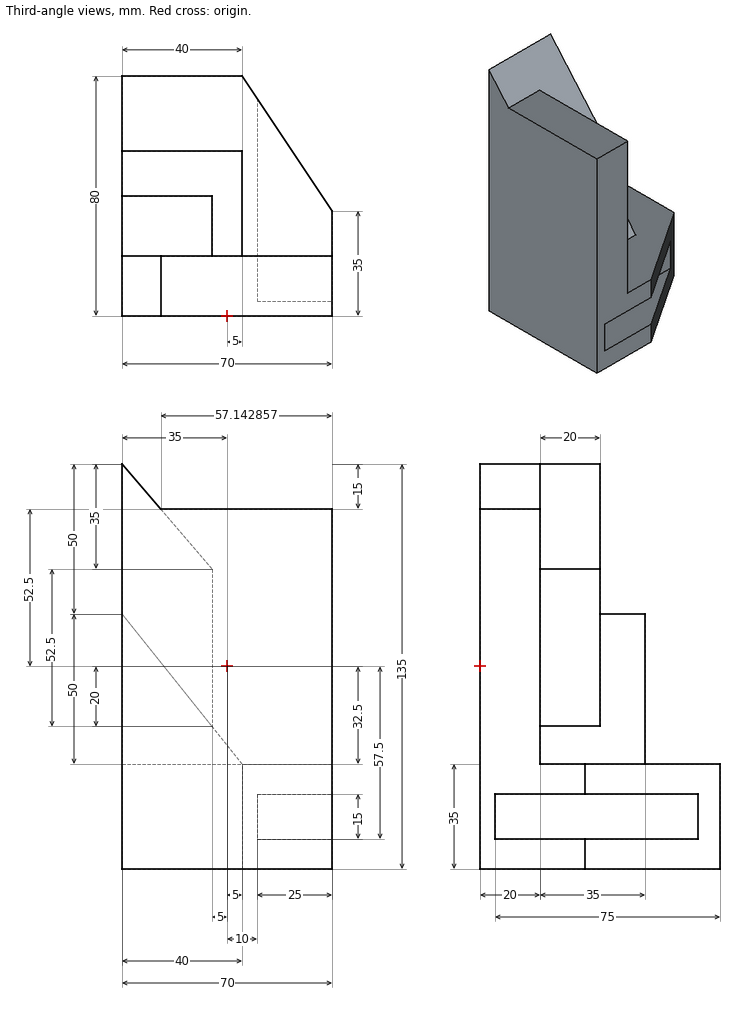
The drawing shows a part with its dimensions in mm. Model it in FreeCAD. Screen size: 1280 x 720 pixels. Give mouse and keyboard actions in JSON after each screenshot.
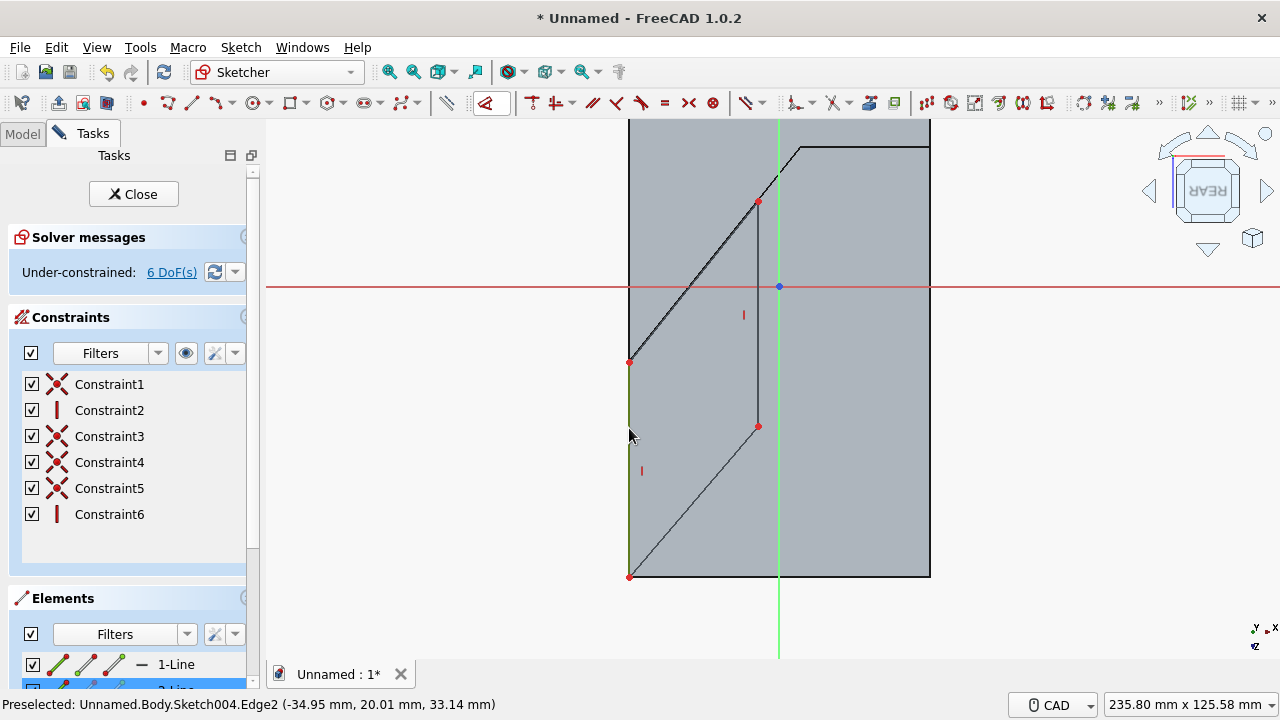
{"action": "left_click", "coordinate": [504, 104]}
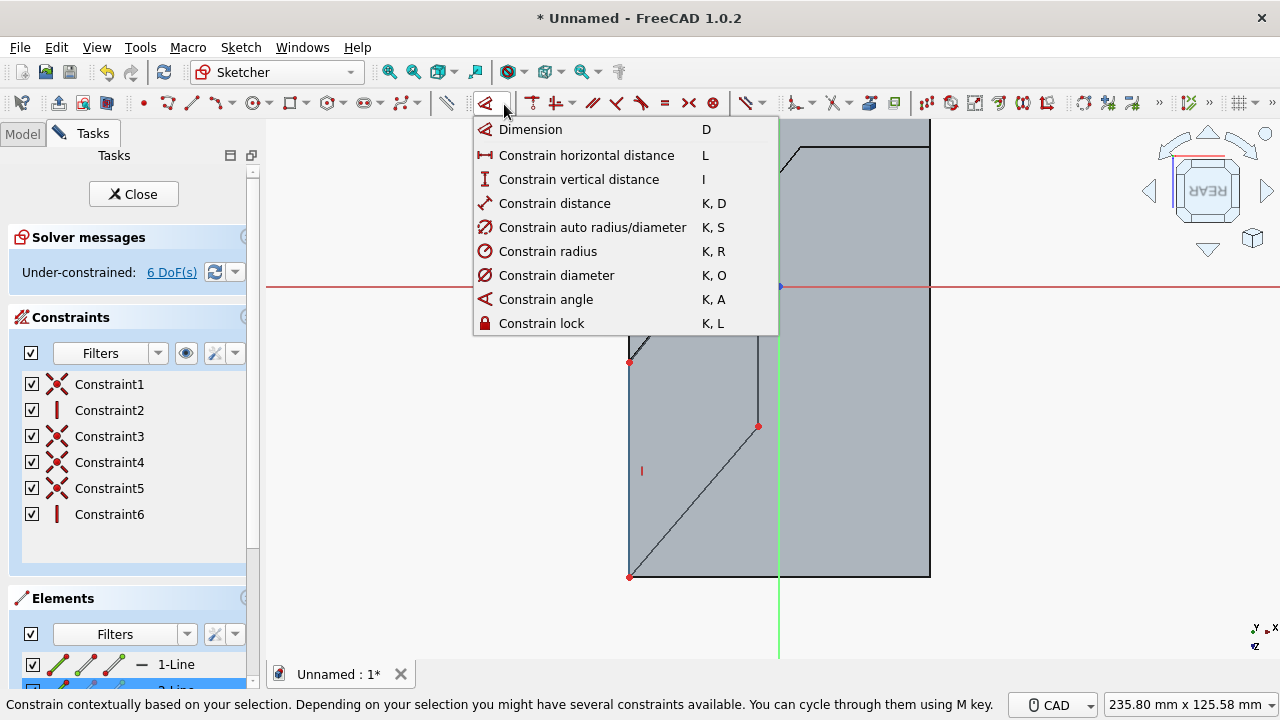
{"action": "left_click", "coordinate": [626, 179]}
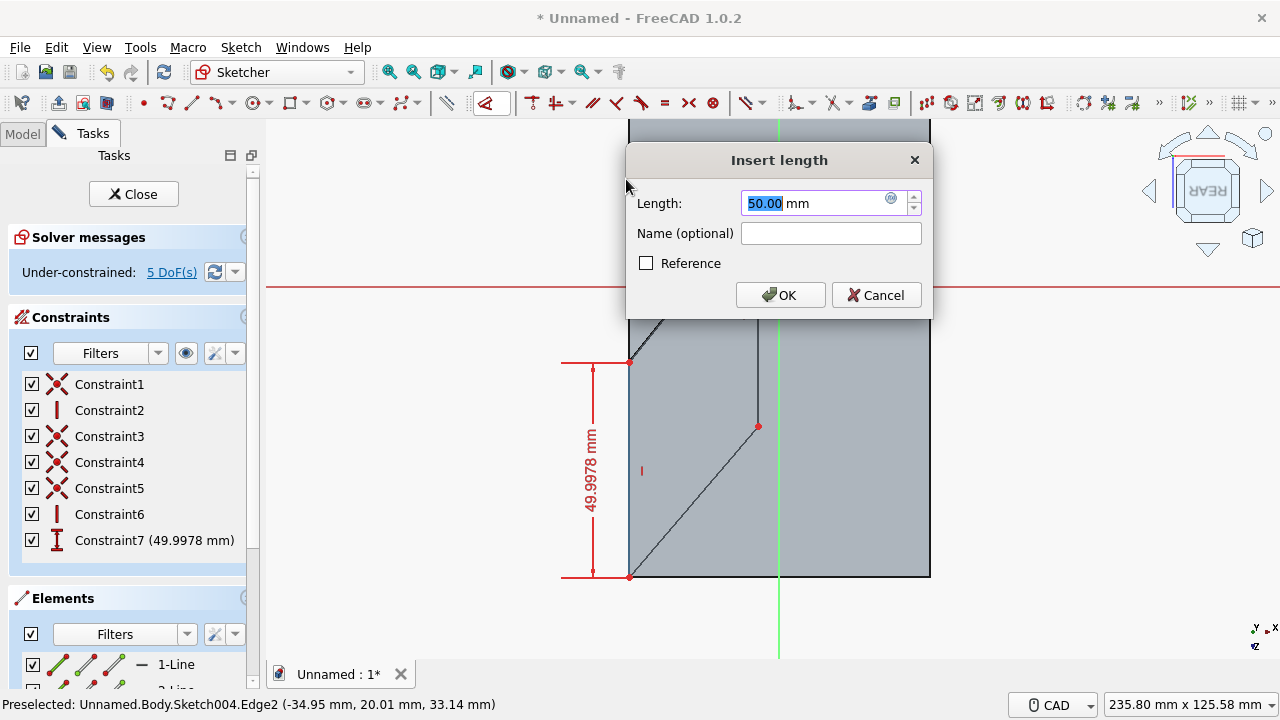
{"action": "type", "text": "50"}
{"action": "key", "text": "Return"}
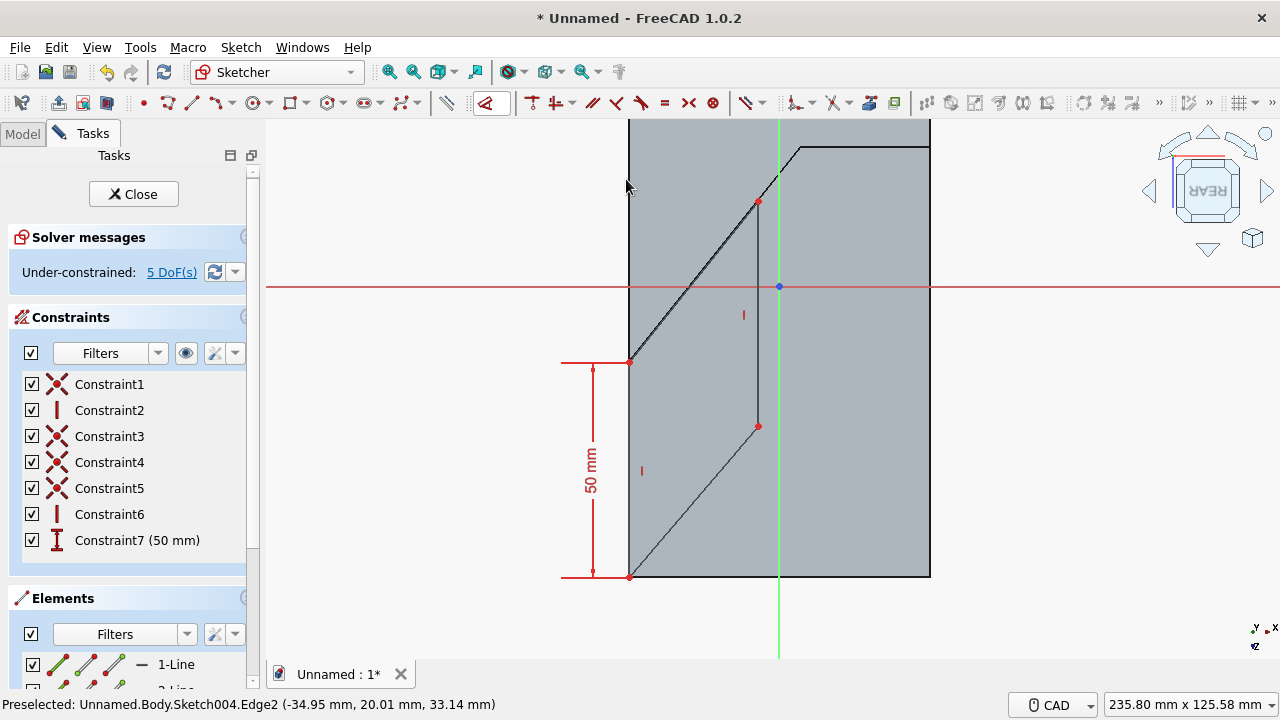
{"action": "scroll", "coordinate": [758, 202], "scroll_direction": "up", "scroll_amount": 4}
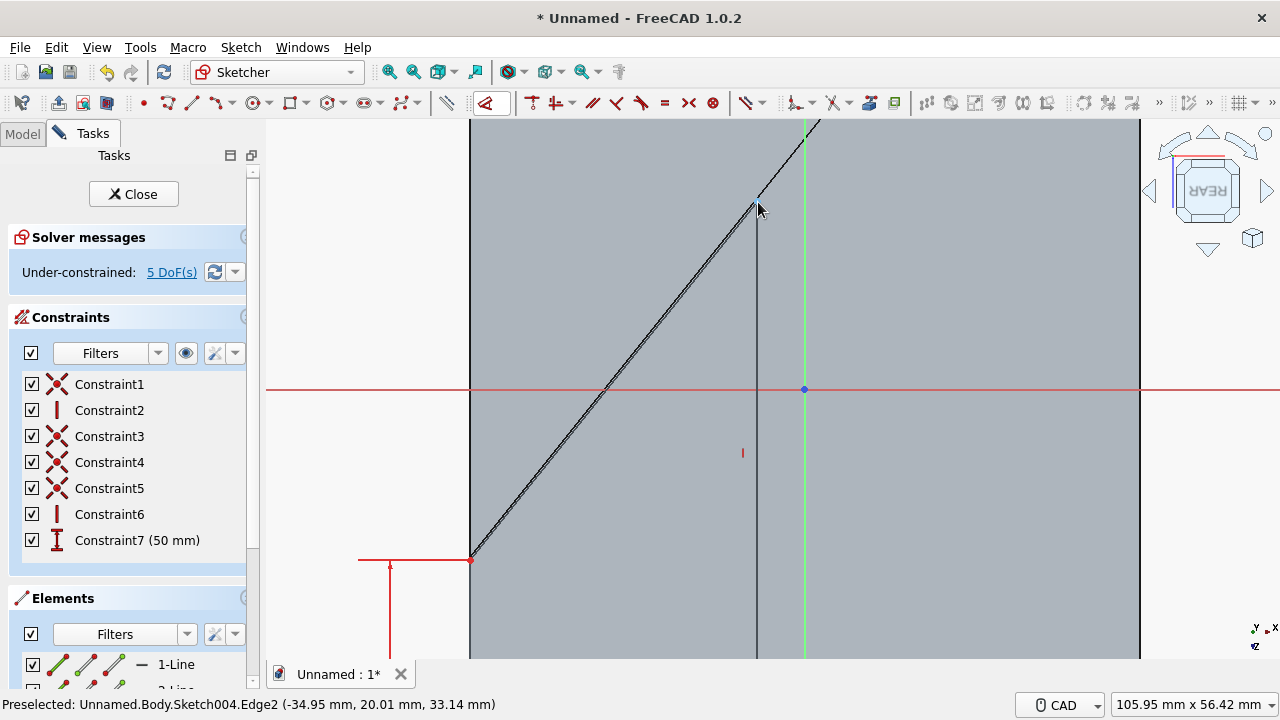
{"action": "left_click", "coordinate": [757, 202]}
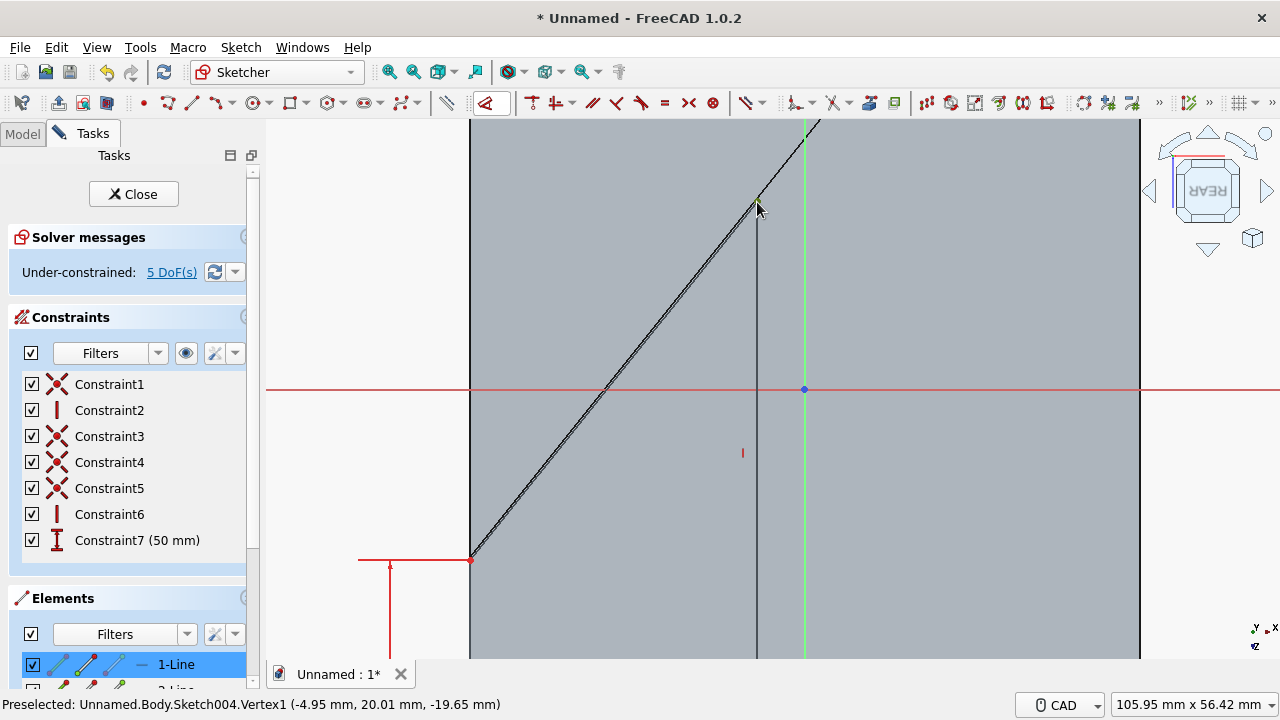
{"action": "left_click", "coordinate": [504, 104]}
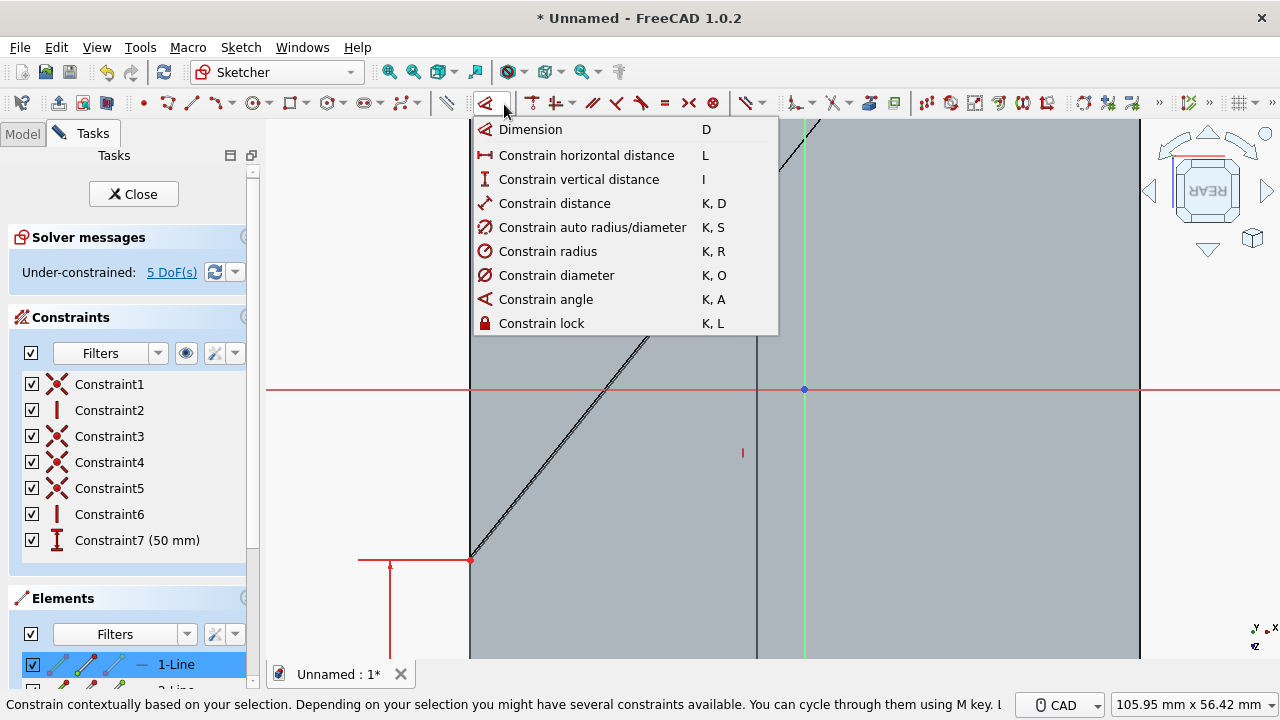
{"action": "left_click", "coordinate": [626, 155]}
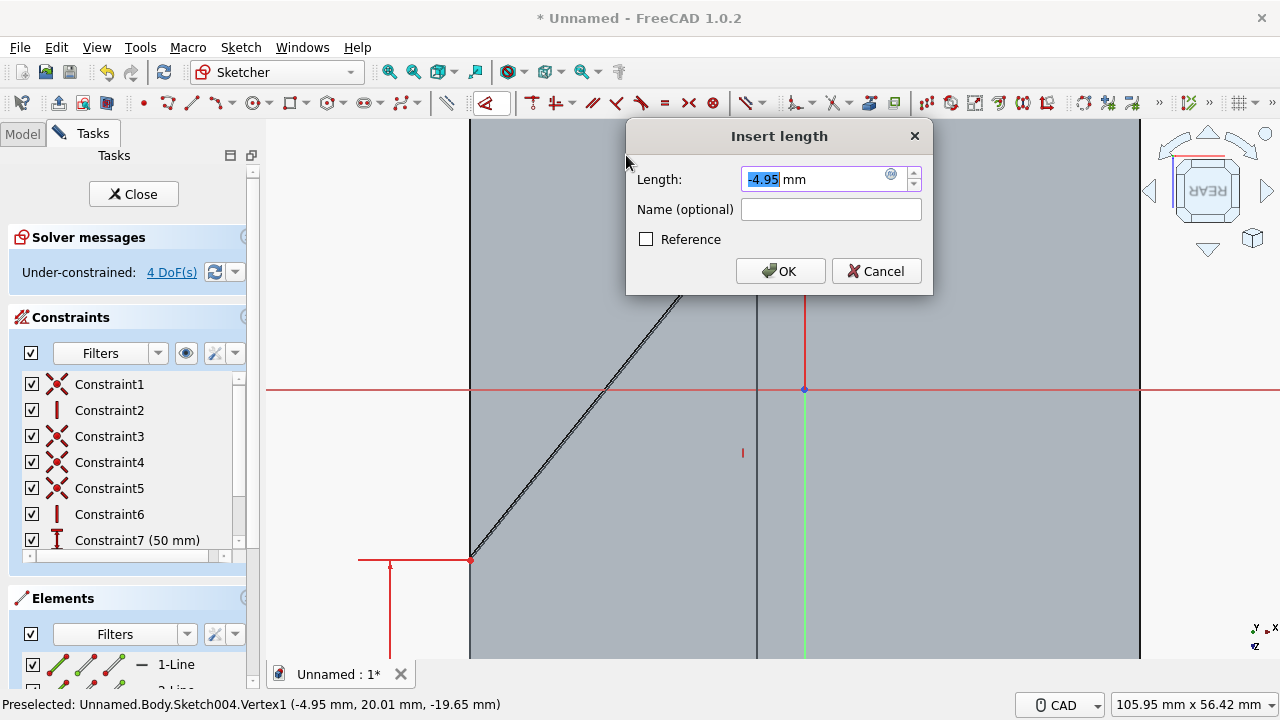
{"action": "type", "text": "-5"}
{"action": "key", "text": "Return"}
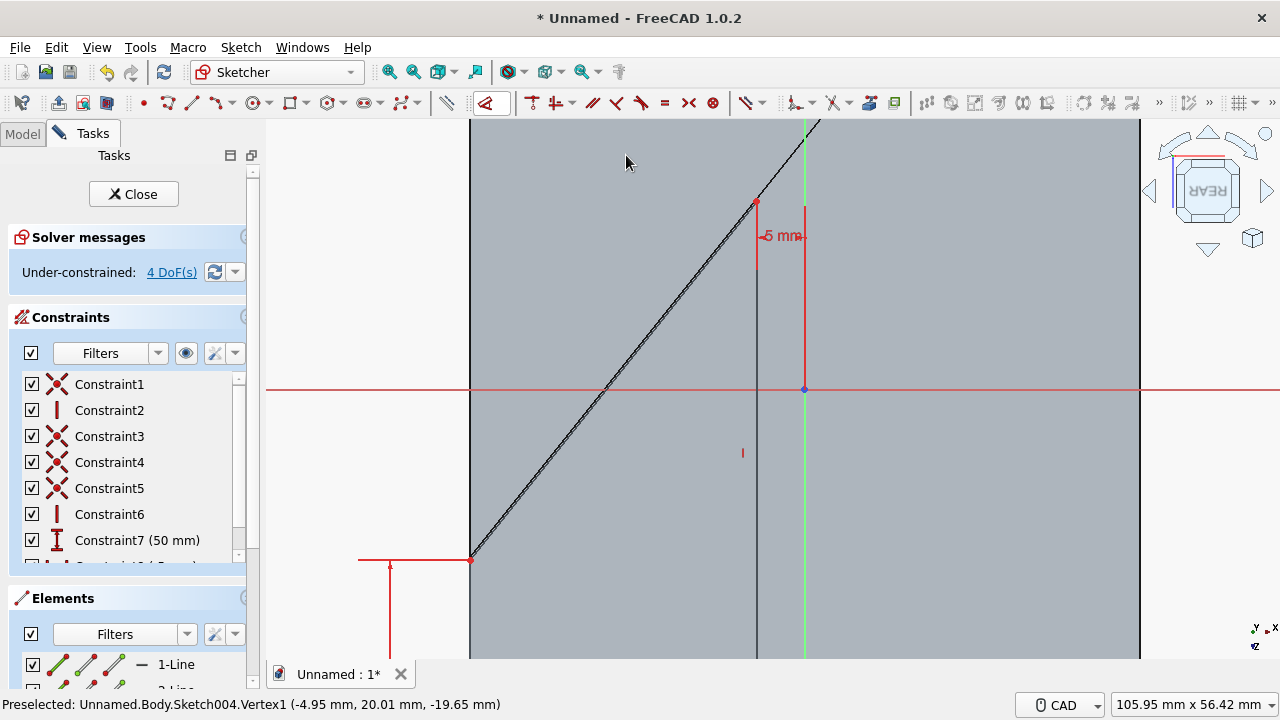
{"action": "left_click", "coordinate": [757, 202]}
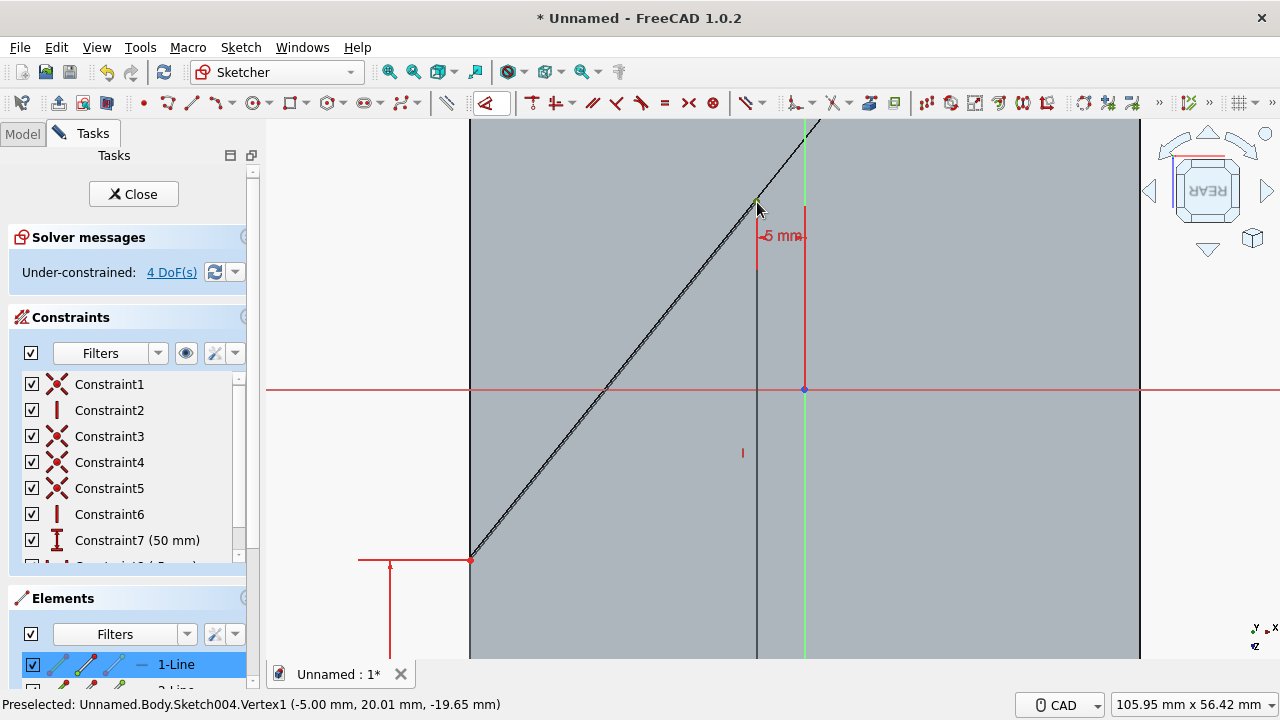
{"action": "left_click", "coordinate": [504, 104]}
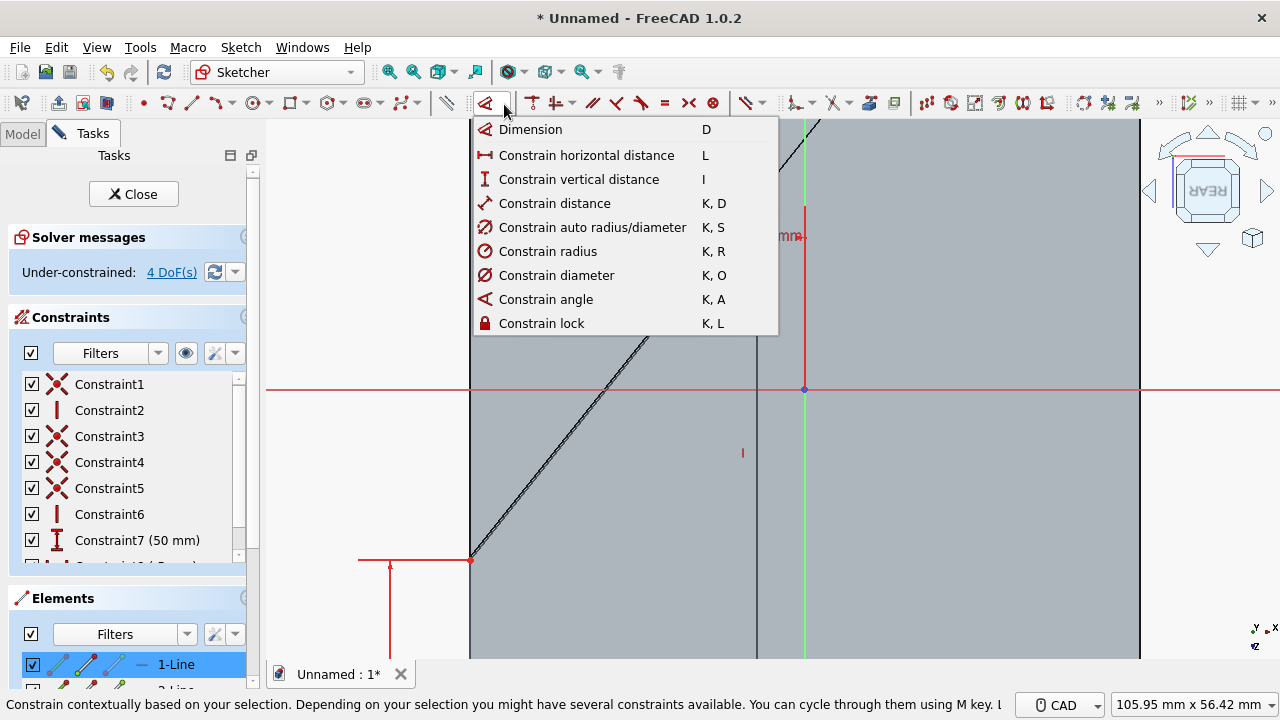
{"action": "left_click", "coordinate": [626, 179]}